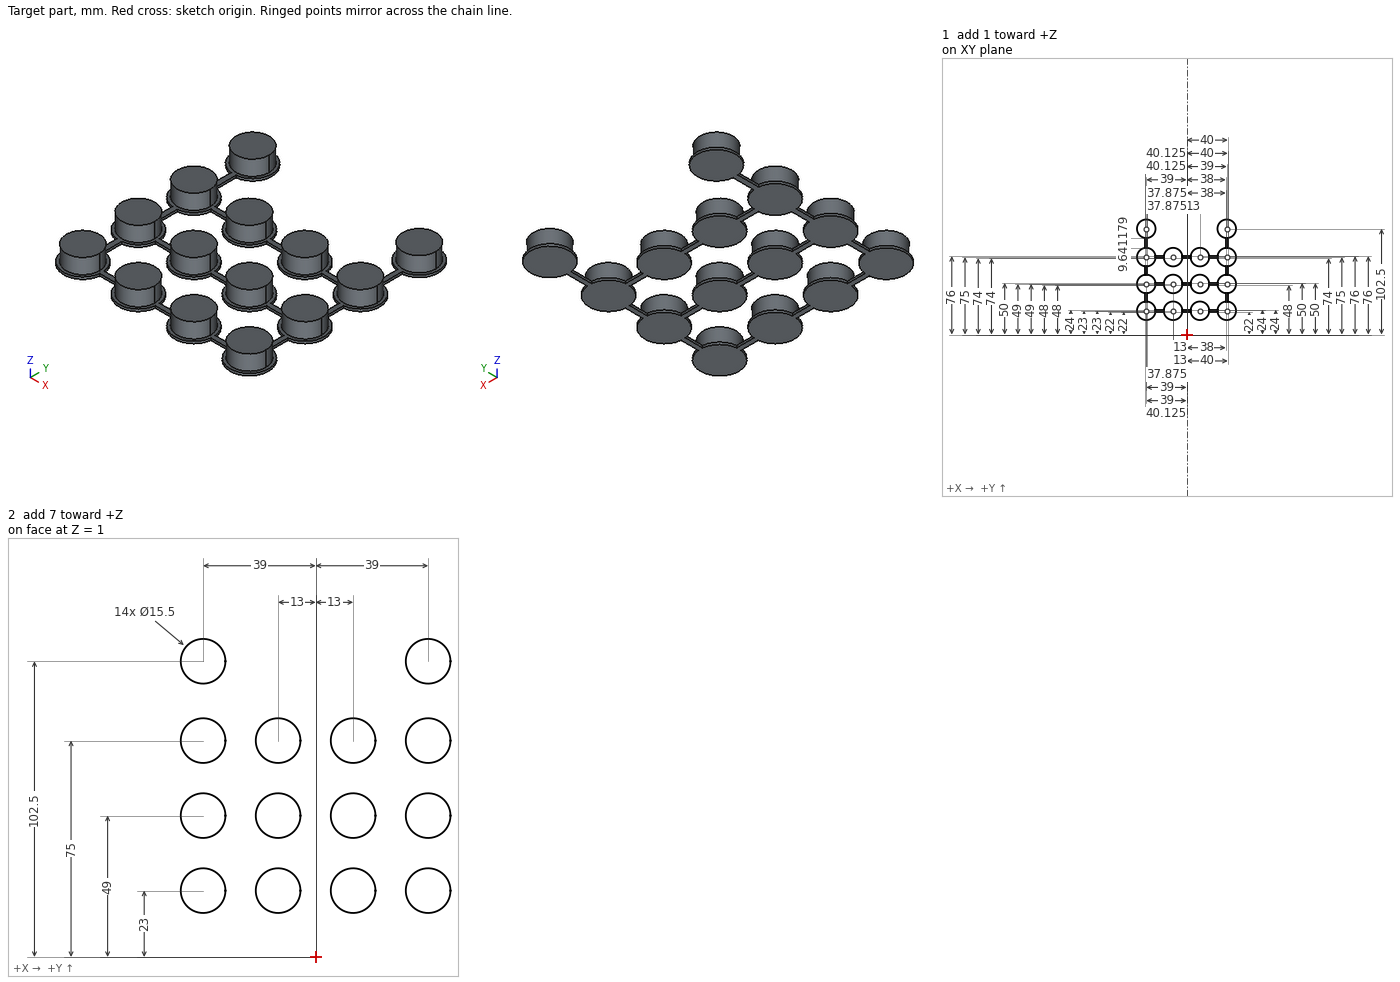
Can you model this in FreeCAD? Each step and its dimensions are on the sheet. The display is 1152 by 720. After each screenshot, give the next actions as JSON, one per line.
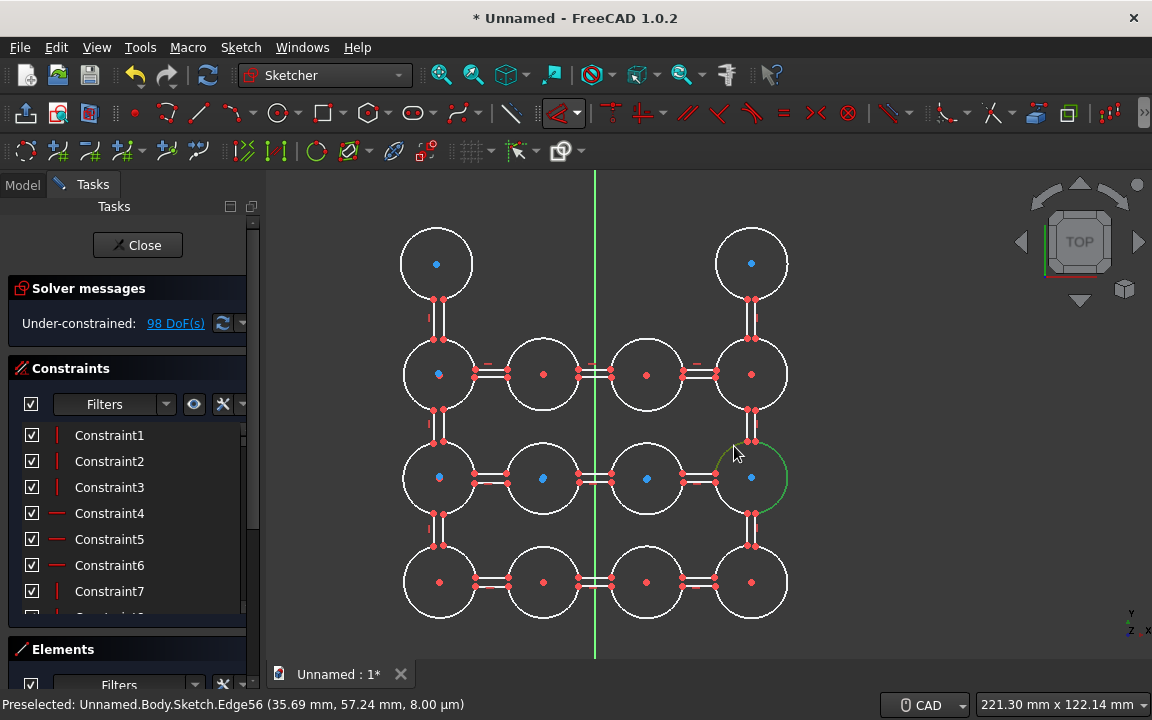
{"action": "left_click", "coordinate": [612, 114]}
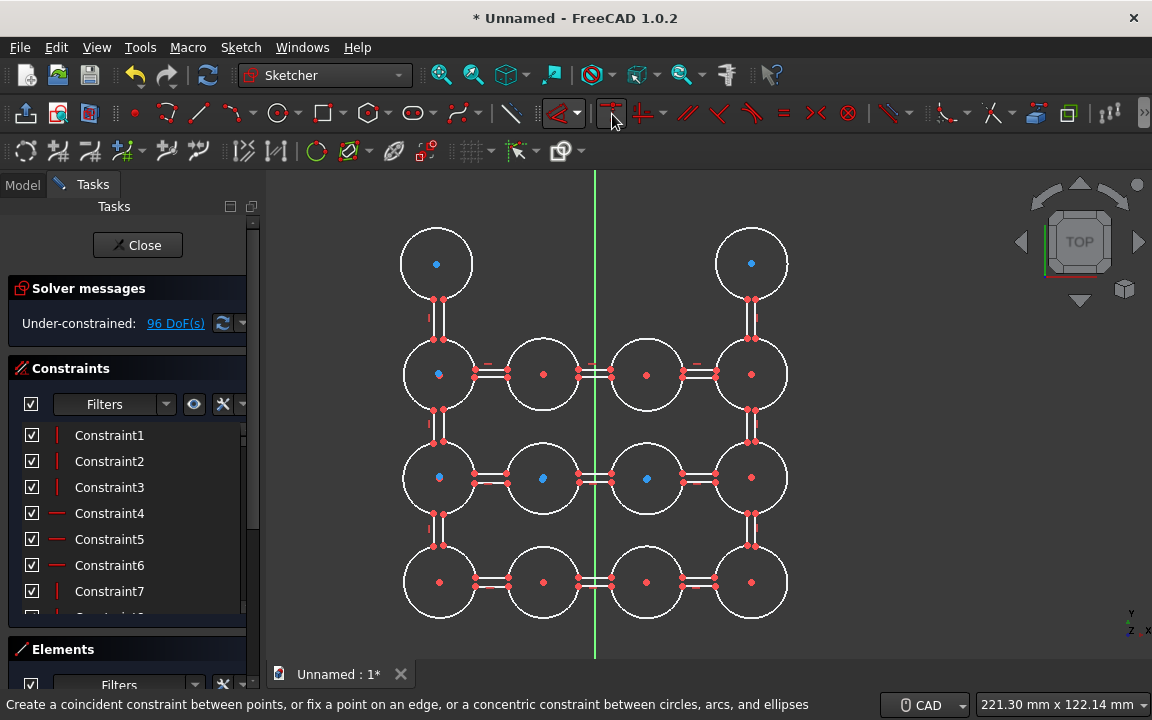
{"action": "left_click", "coordinate": [627, 508]}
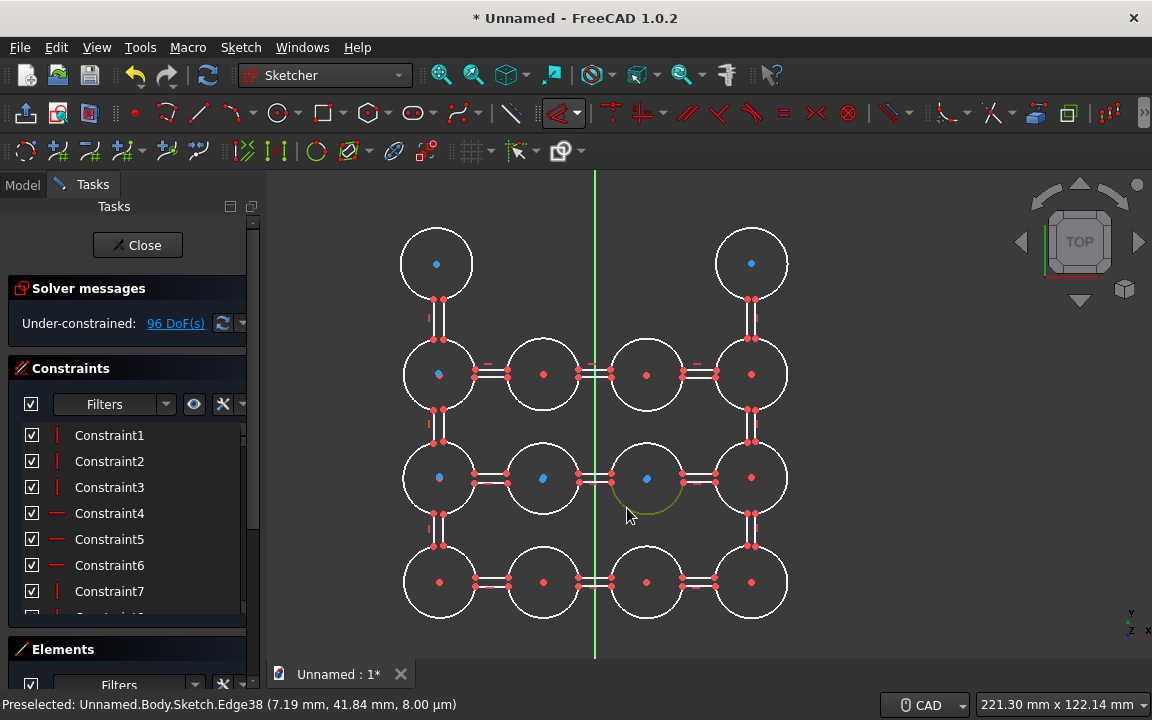
{"action": "left_click", "coordinate": [666, 449]}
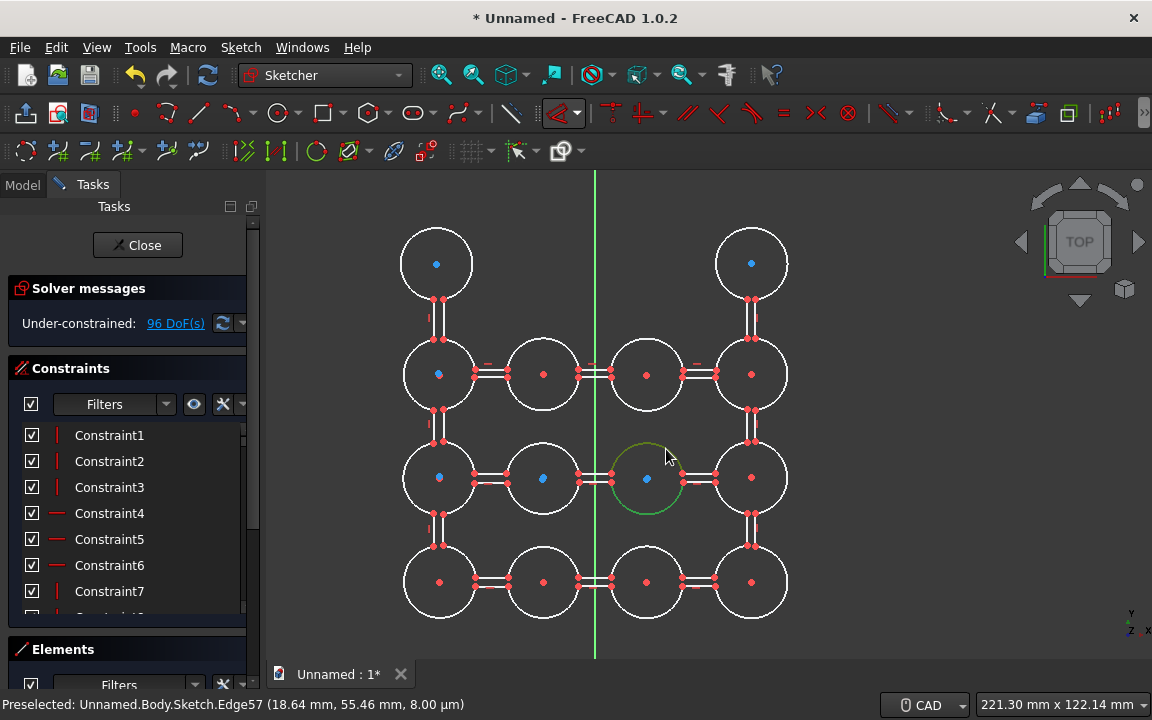
{"action": "left_click", "coordinate": [612, 114]}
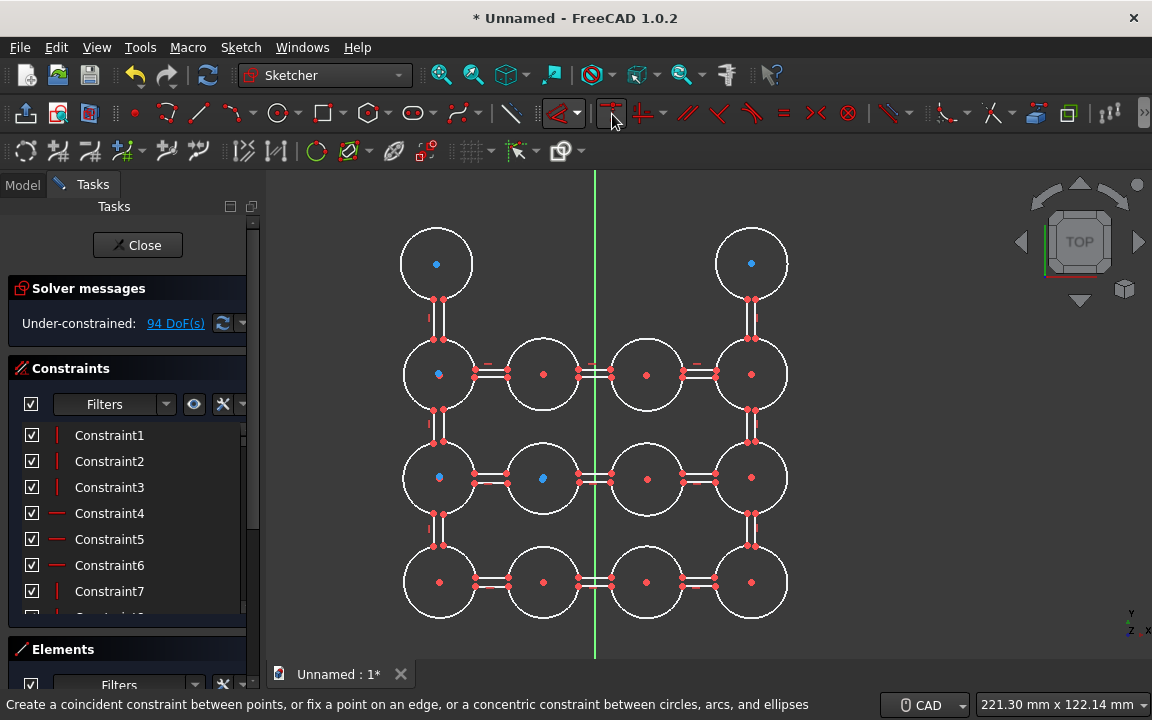
{"action": "left_click", "coordinate": [524, 508]}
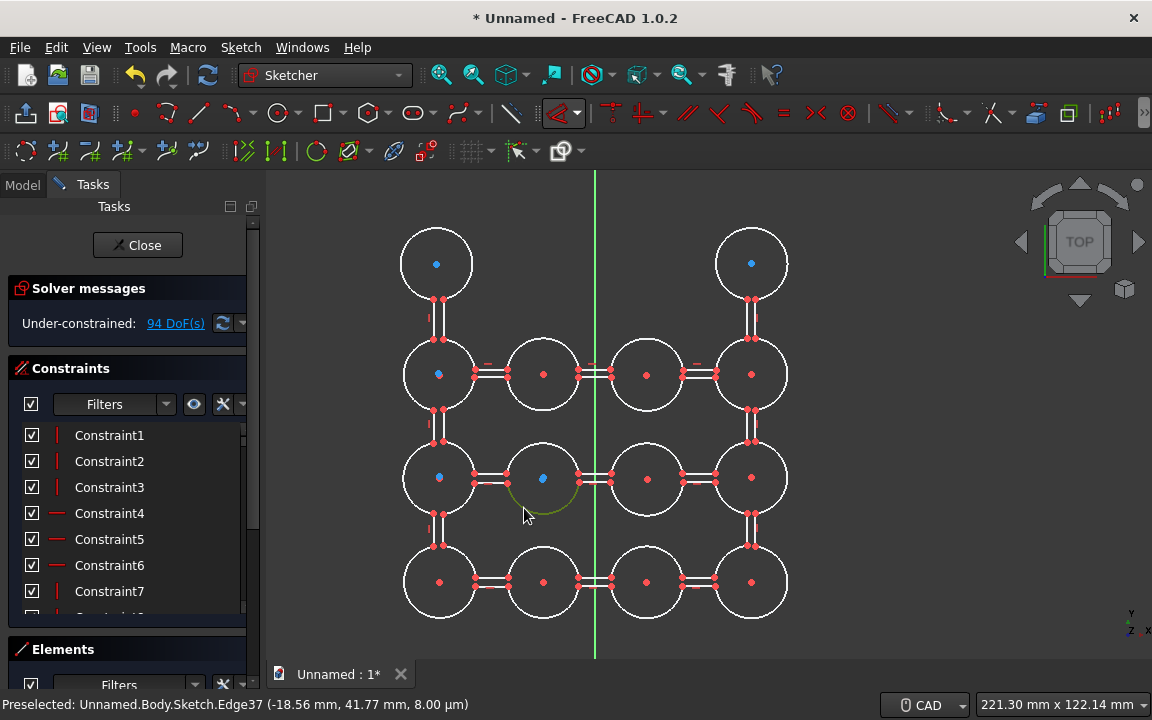
{"action": "left_click", "coordinate": [562, 449]}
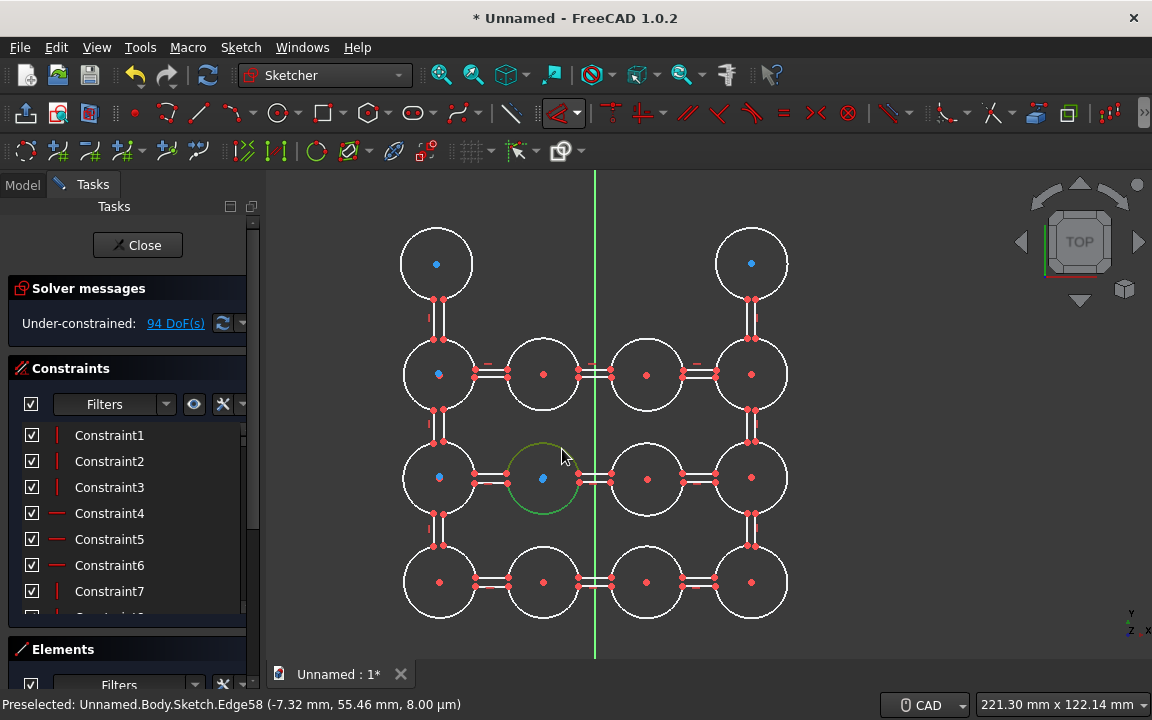
{"action": "left_click", "coordinate": [612, 114]}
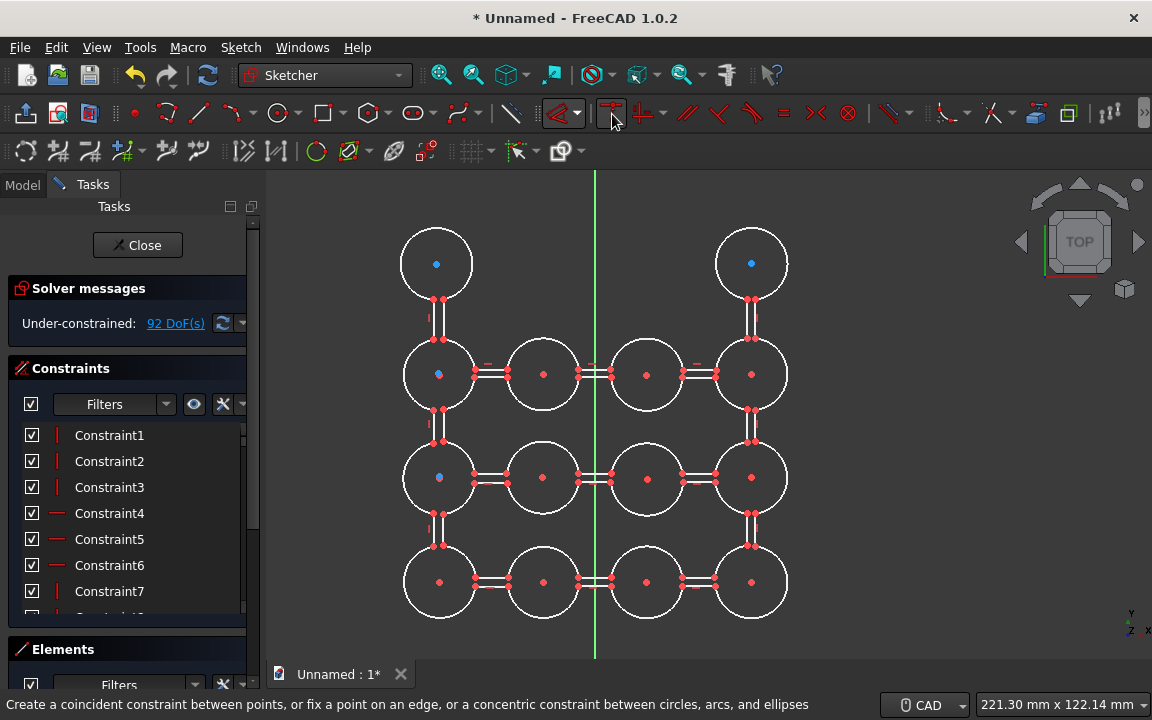
{"action": "left_click", "coordinate": [409, 459]}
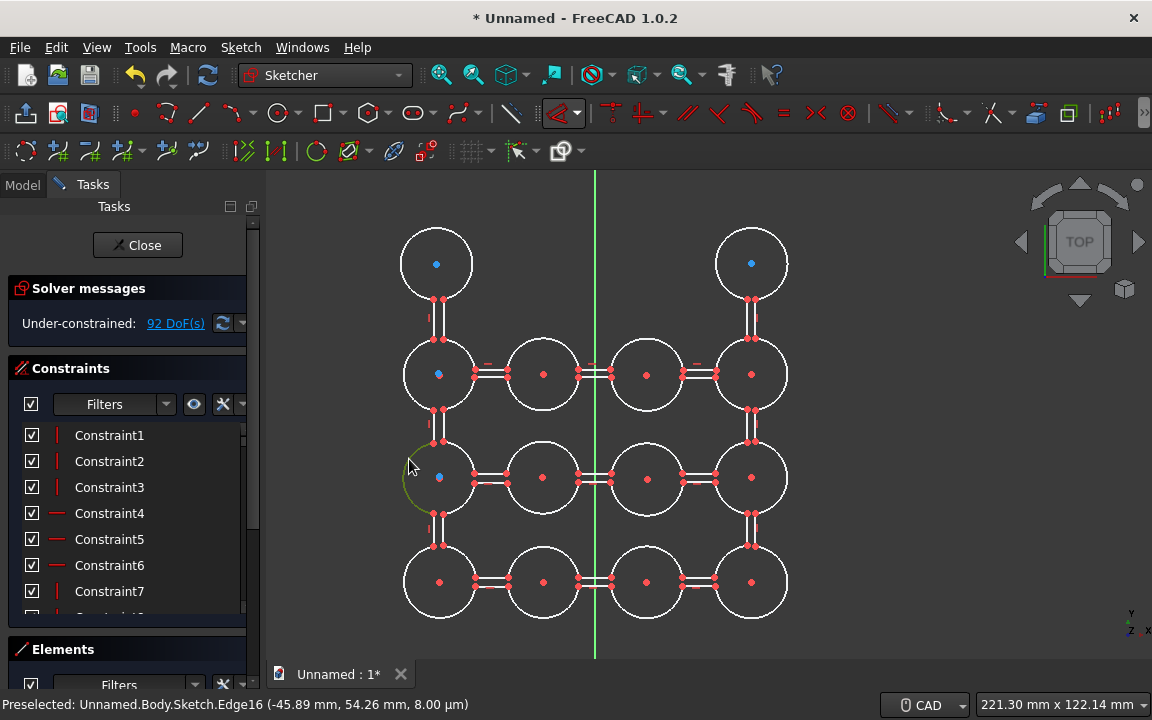
{"action": "left_click", "coordinate": [470, 460]}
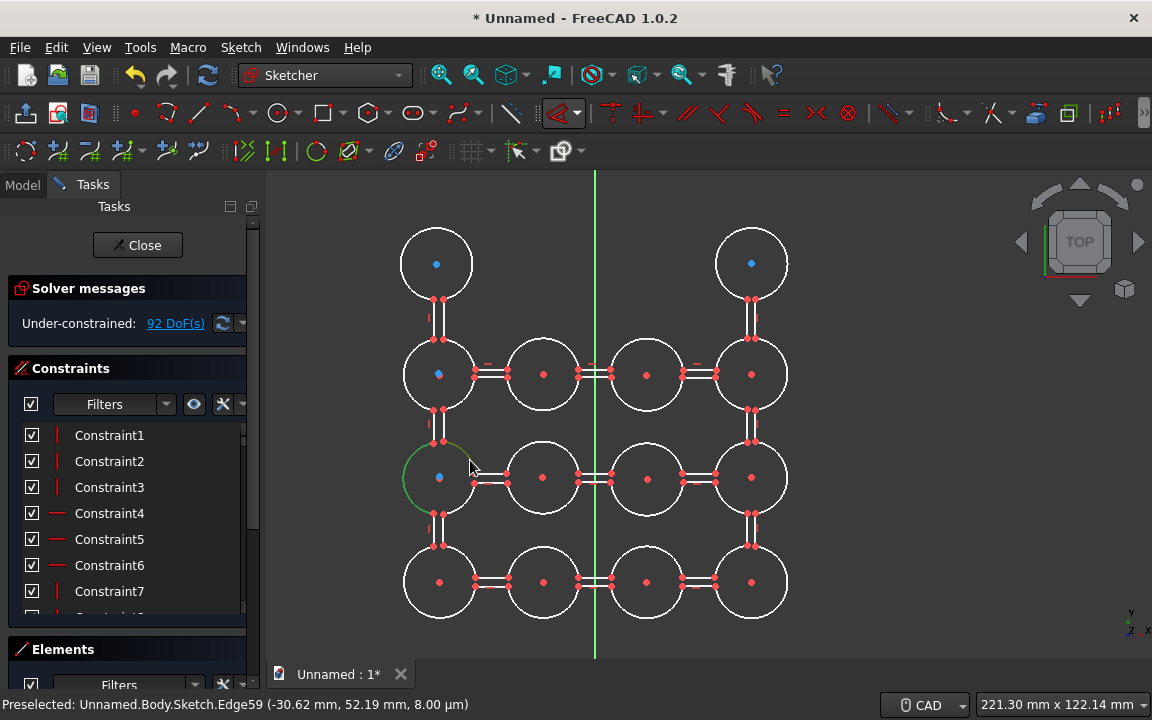
{"action": "left_click", "coordinate": [612, 114]}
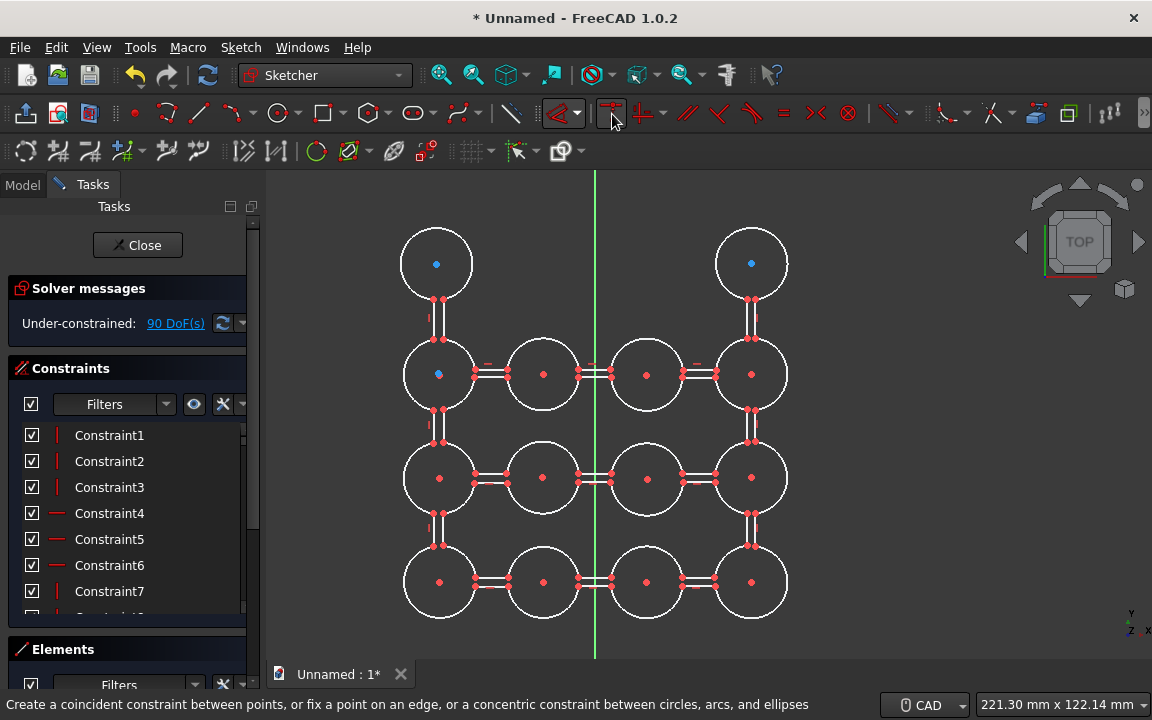
{"action": "left_click", "coordinate": [409, 356]}